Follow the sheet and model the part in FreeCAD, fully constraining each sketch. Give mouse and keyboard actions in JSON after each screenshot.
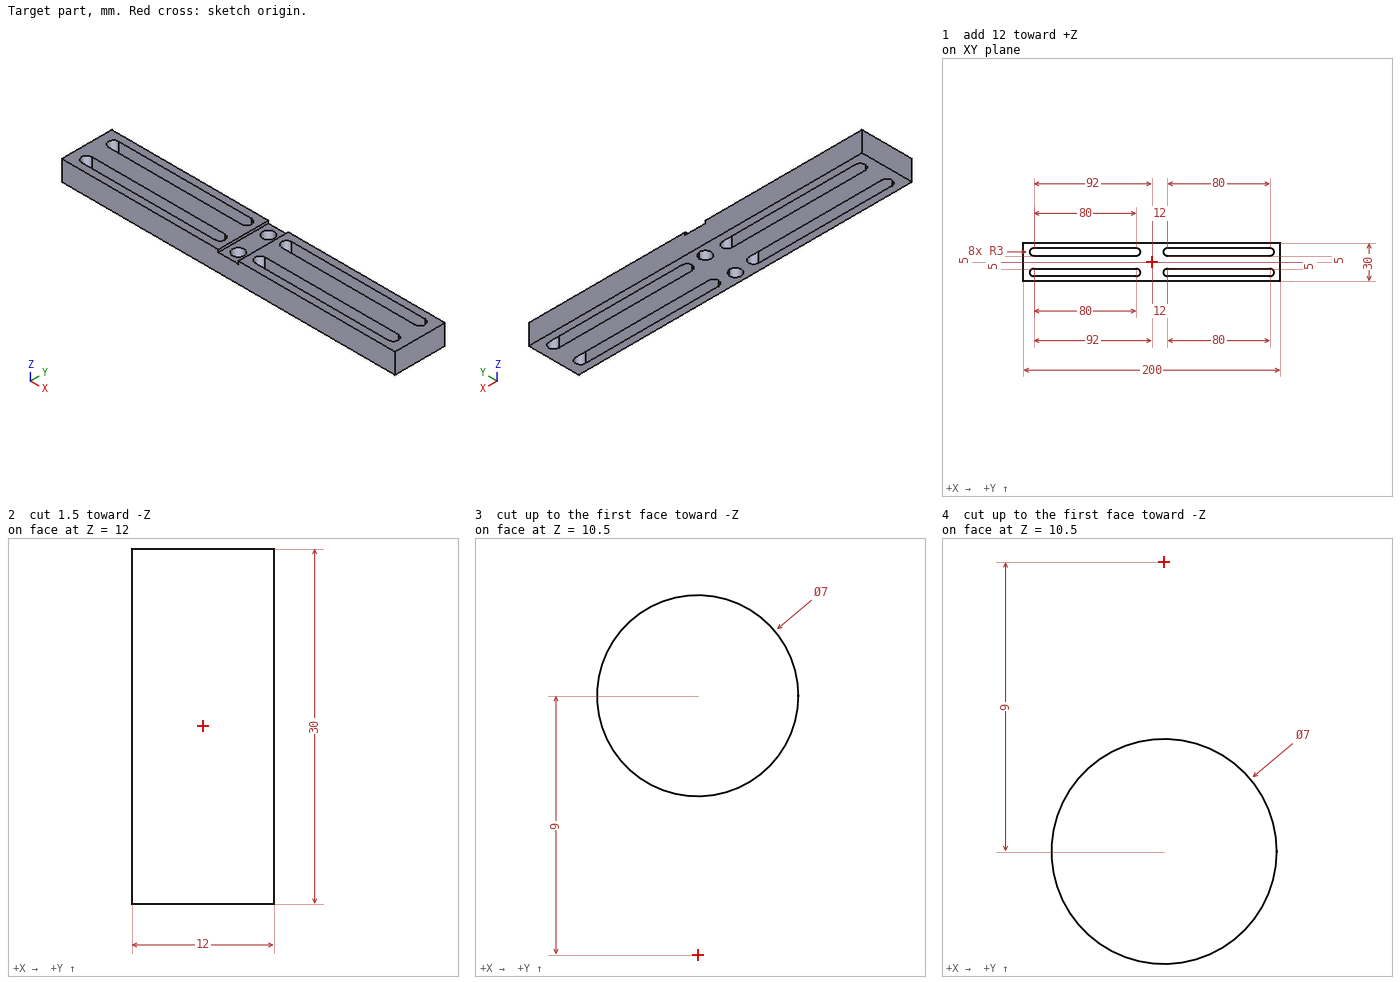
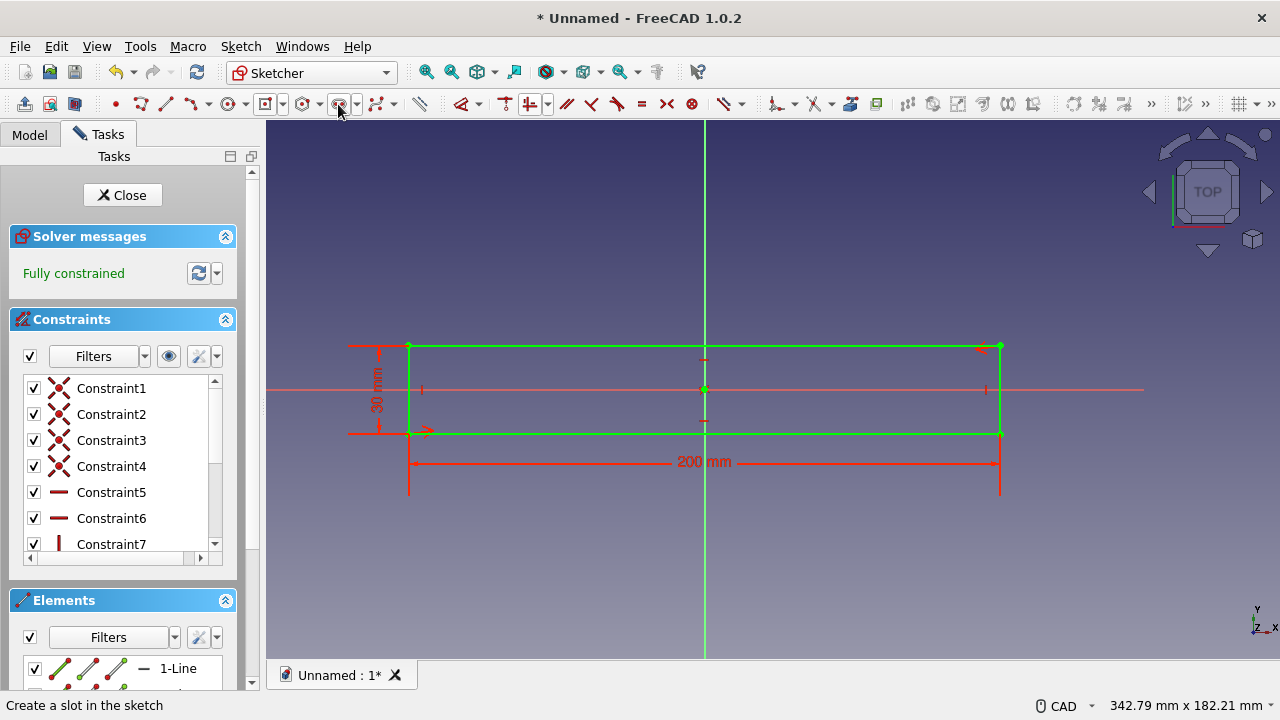
{"action": "scroll", "coordinate": [432, 414], "scroll_direction": "up", "scroll_amount": 5}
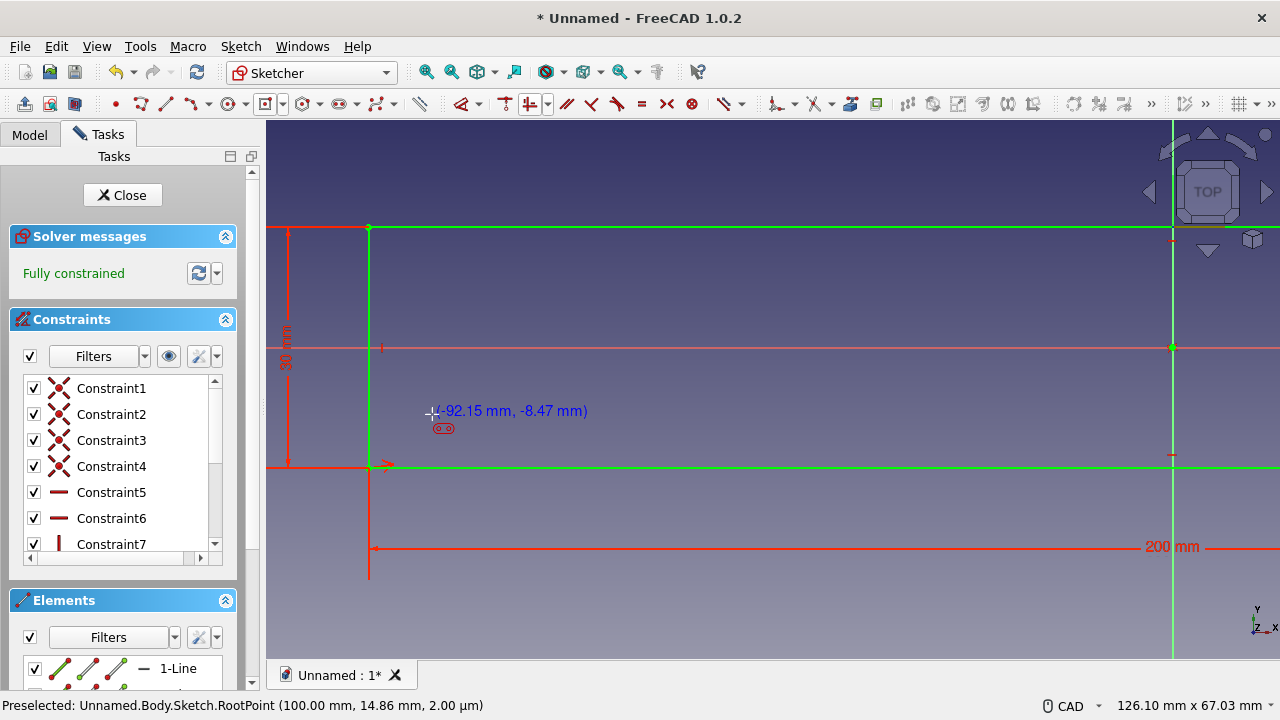
{"action": "left_click", "coordinate": [433, 412]}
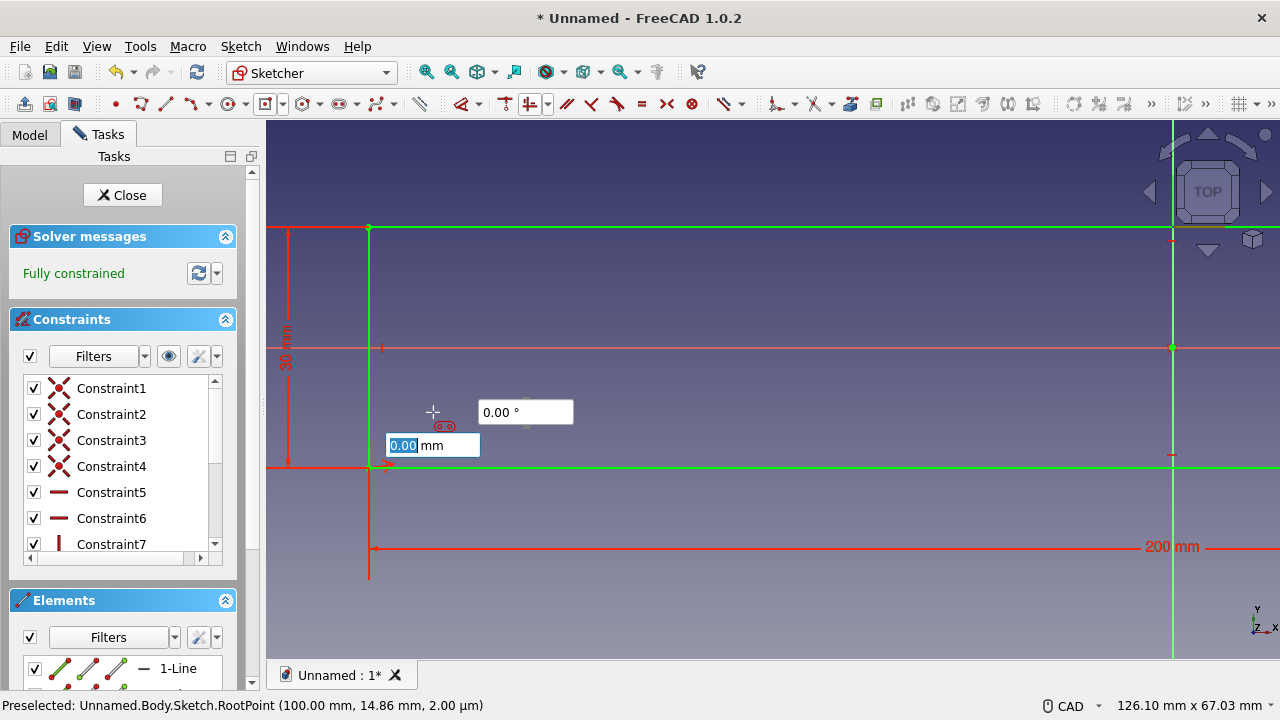
{"action": "left_click", "coordinate": [1076, 412]}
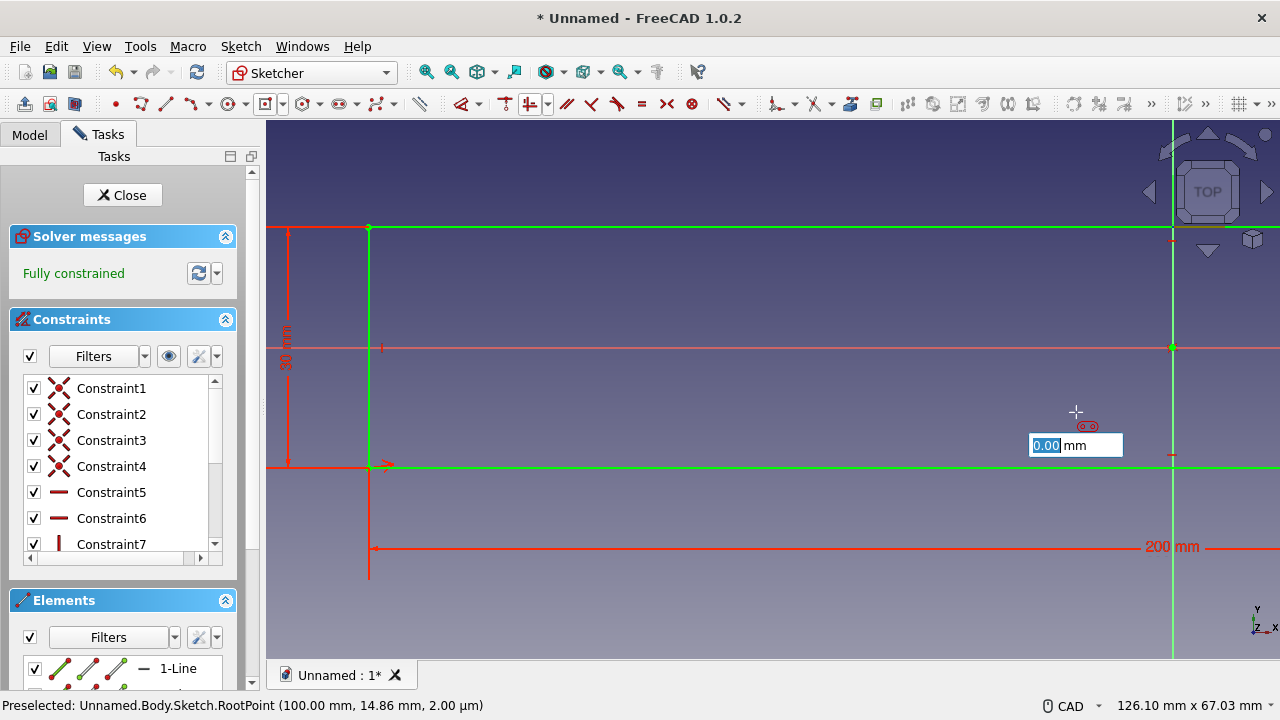
{"action": "left_click", "coordinate": [755, 436]}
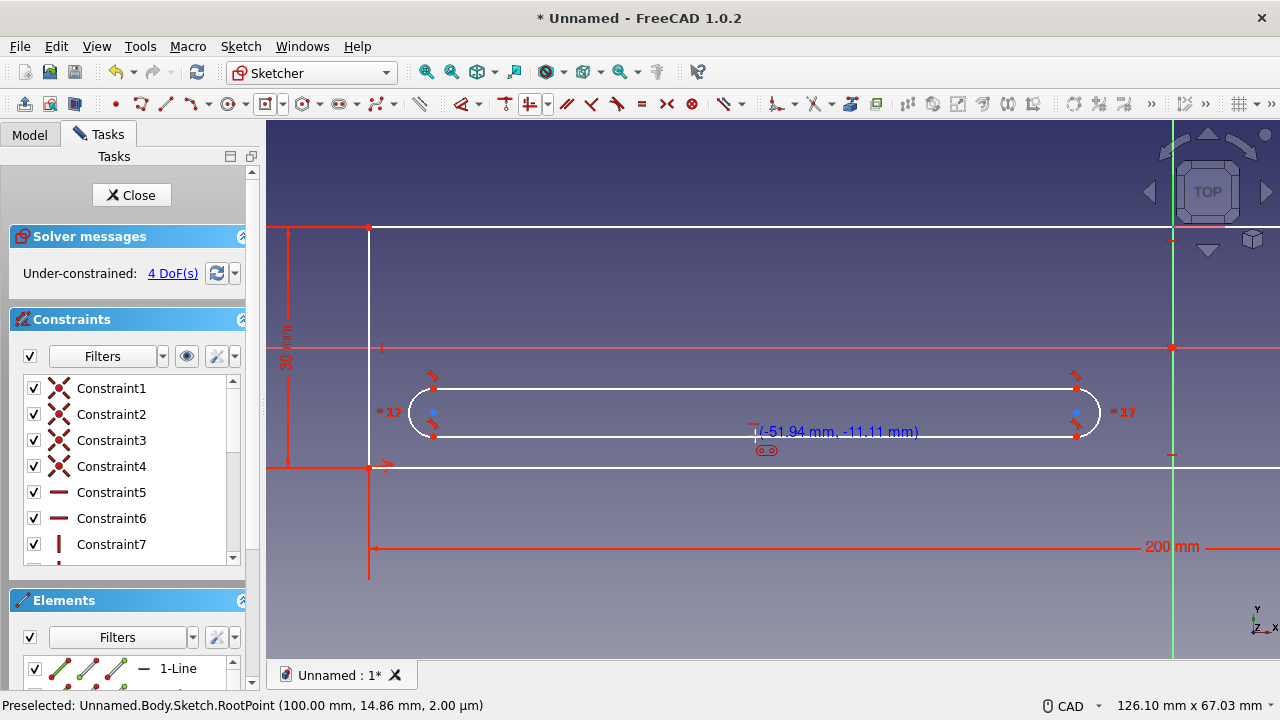
{"action": "scroll", "coordinate": [432, 414], "scroll_direction": "down", "scroll_amount": 5}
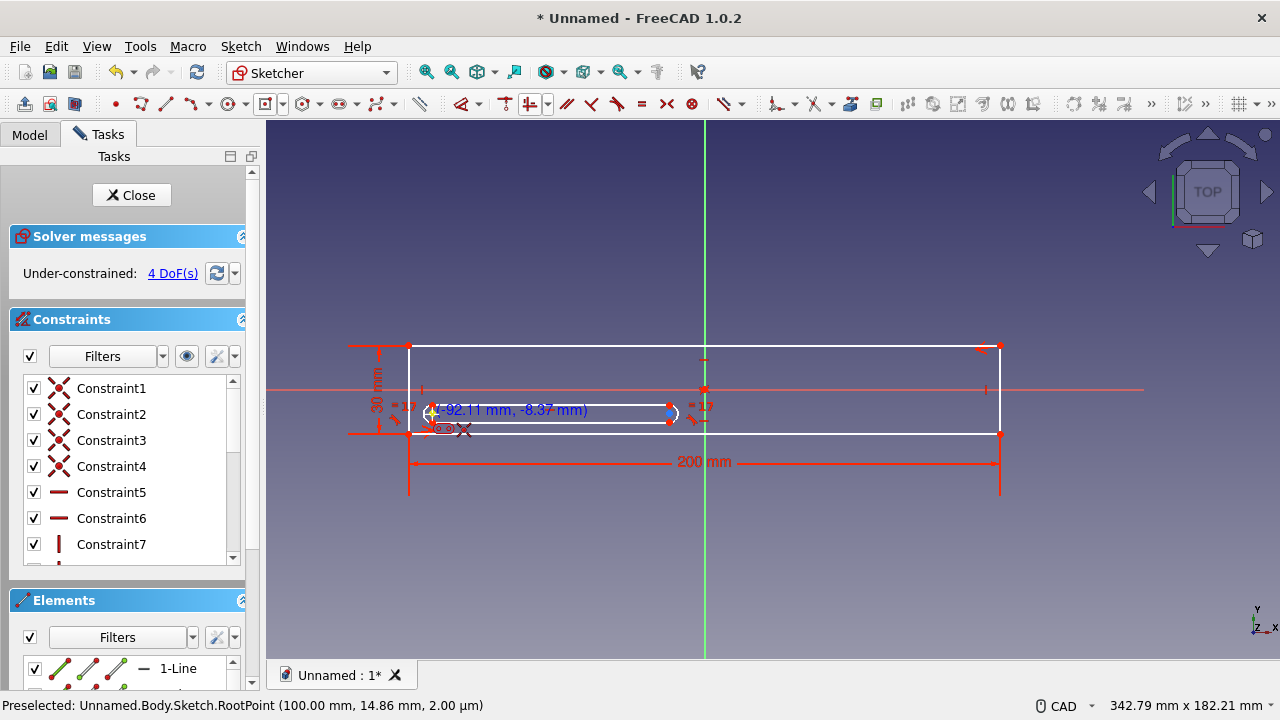
{"action": "scroll", "coordinate": [740, 414], "scroll_direction": "up", "scroll_amount": 5}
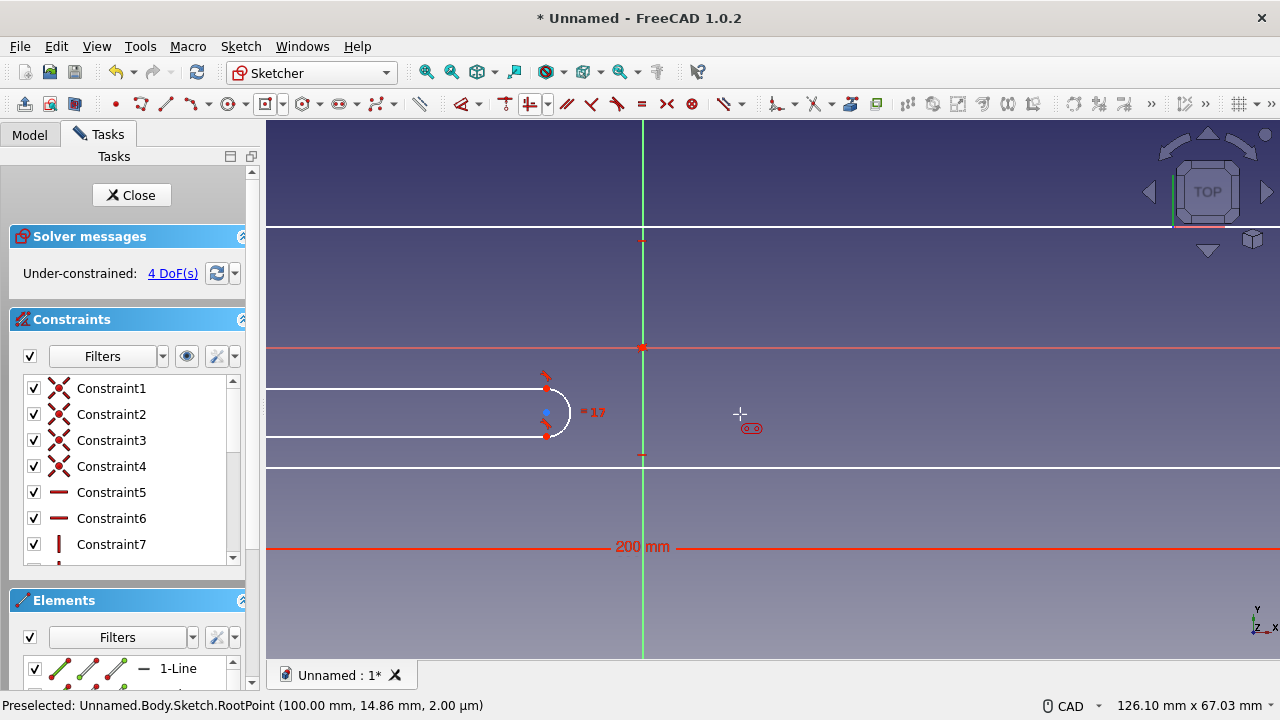
{"action": "left_click", "coordinate": [739, 412]}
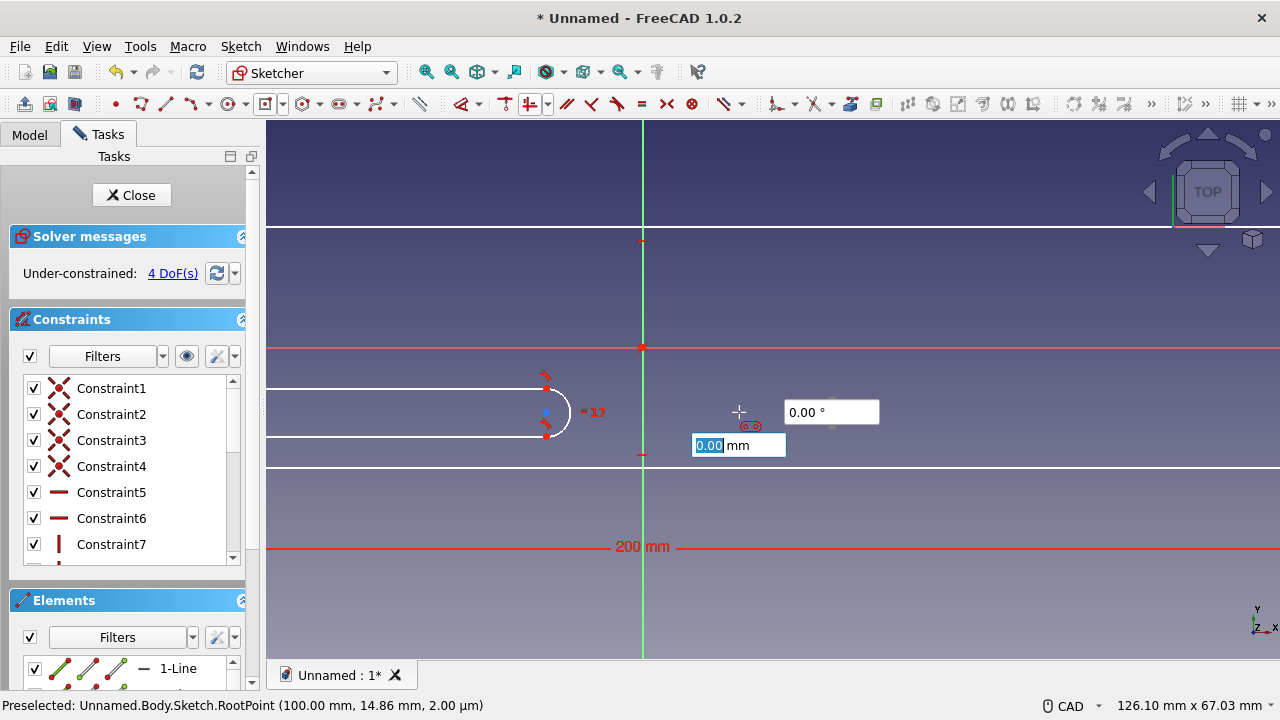
{"action": "scroll", "coordinate": [740, 414], "scroll_direction": "down", "scroll_amount": 5}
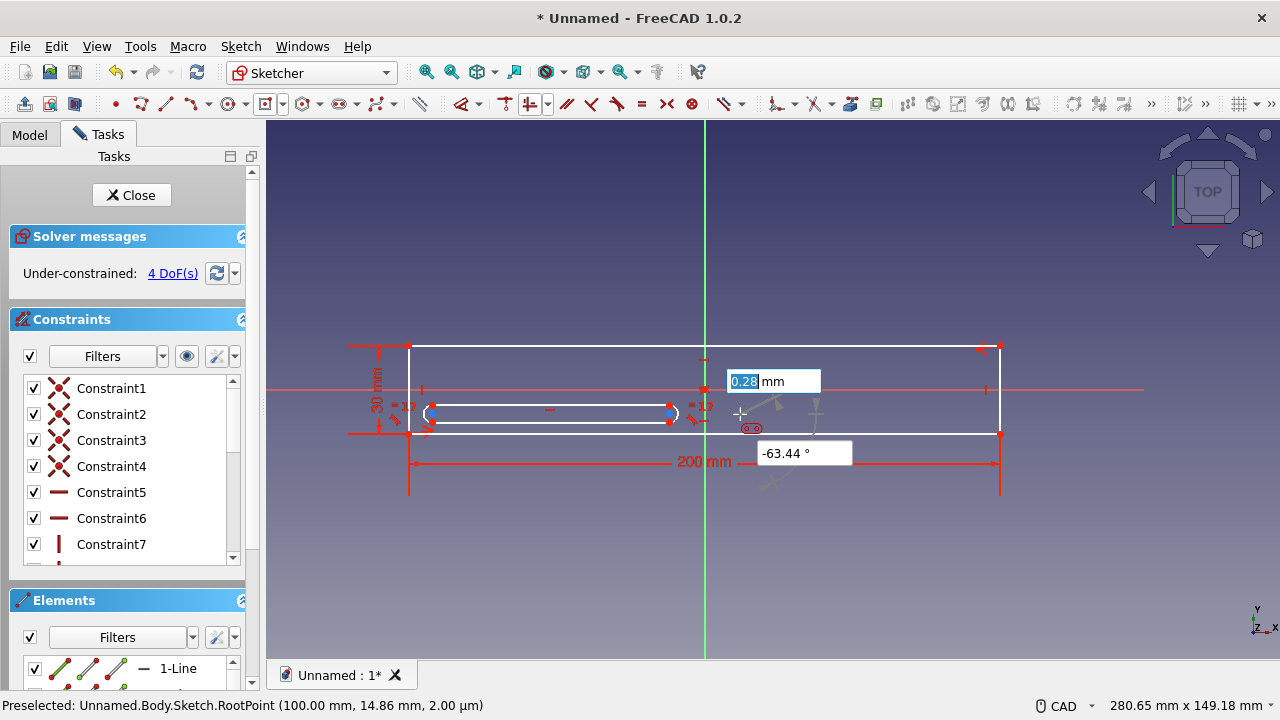
{"action": "left_click", "coordinate": [977, 414]}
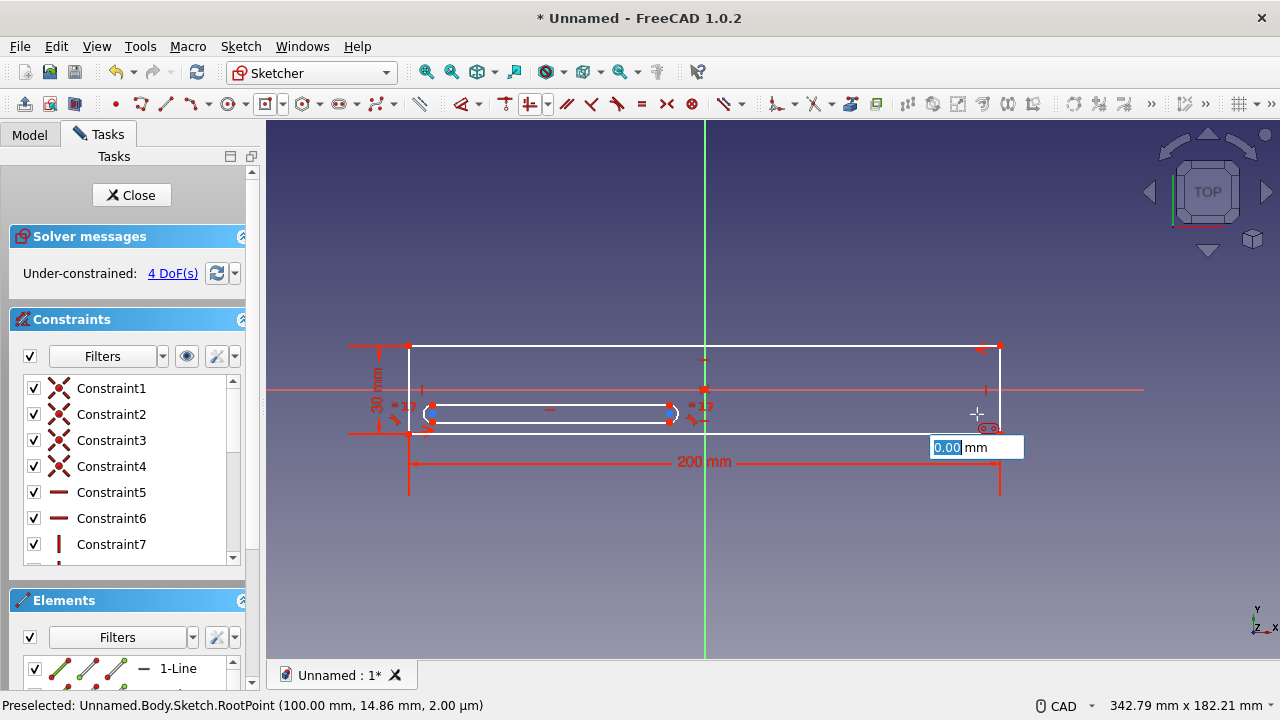
{"action": "scroll", "coordinate": [858, 405], "scroll_direction": "up", "scroll_amount": 3}